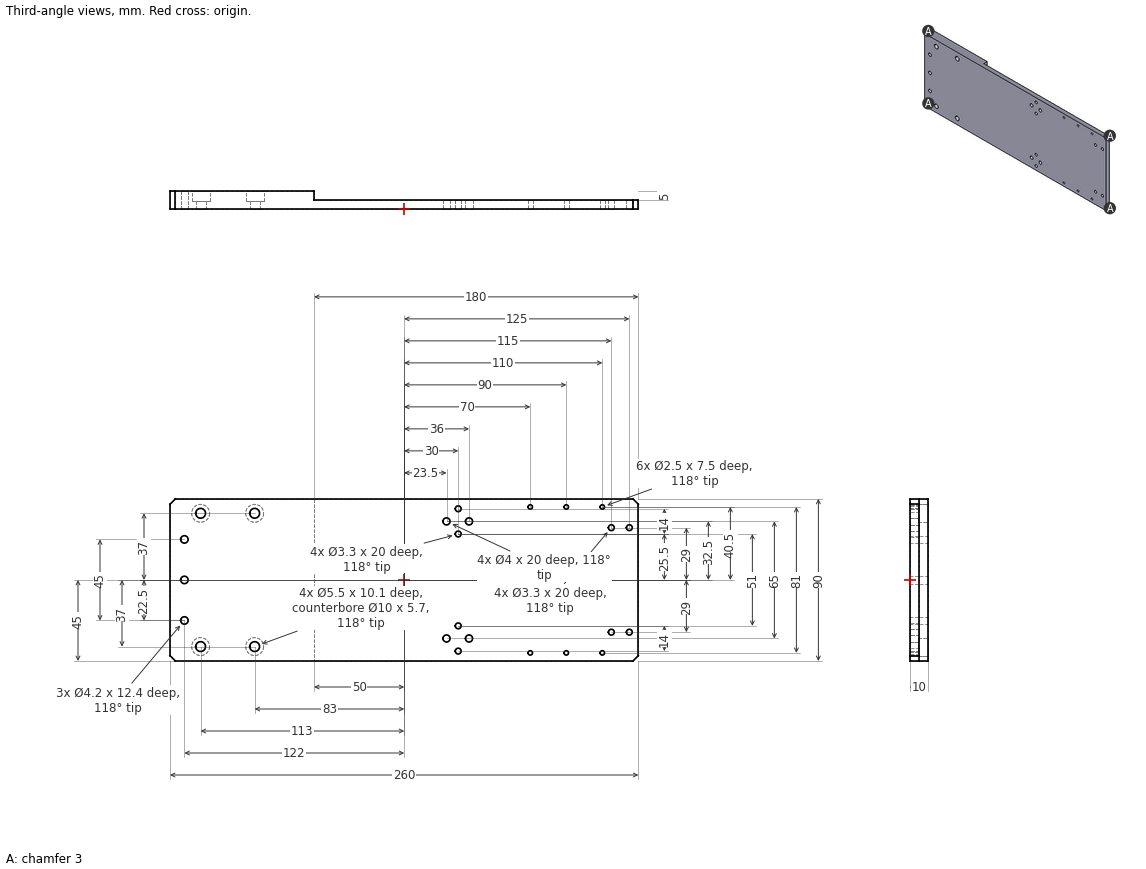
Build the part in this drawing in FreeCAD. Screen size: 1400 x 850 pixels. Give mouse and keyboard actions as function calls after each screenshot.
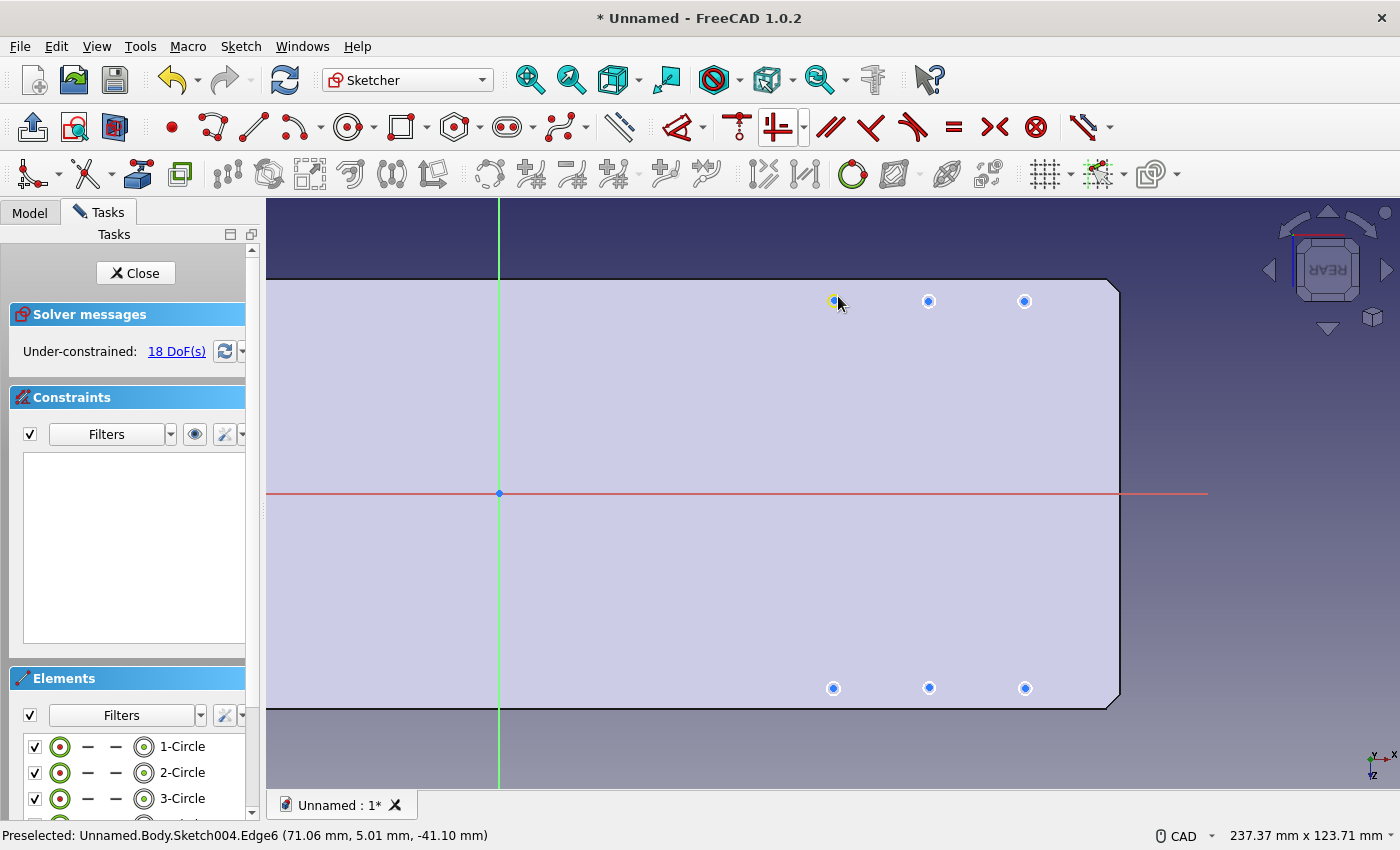
scroll(1030, 684, up, 4)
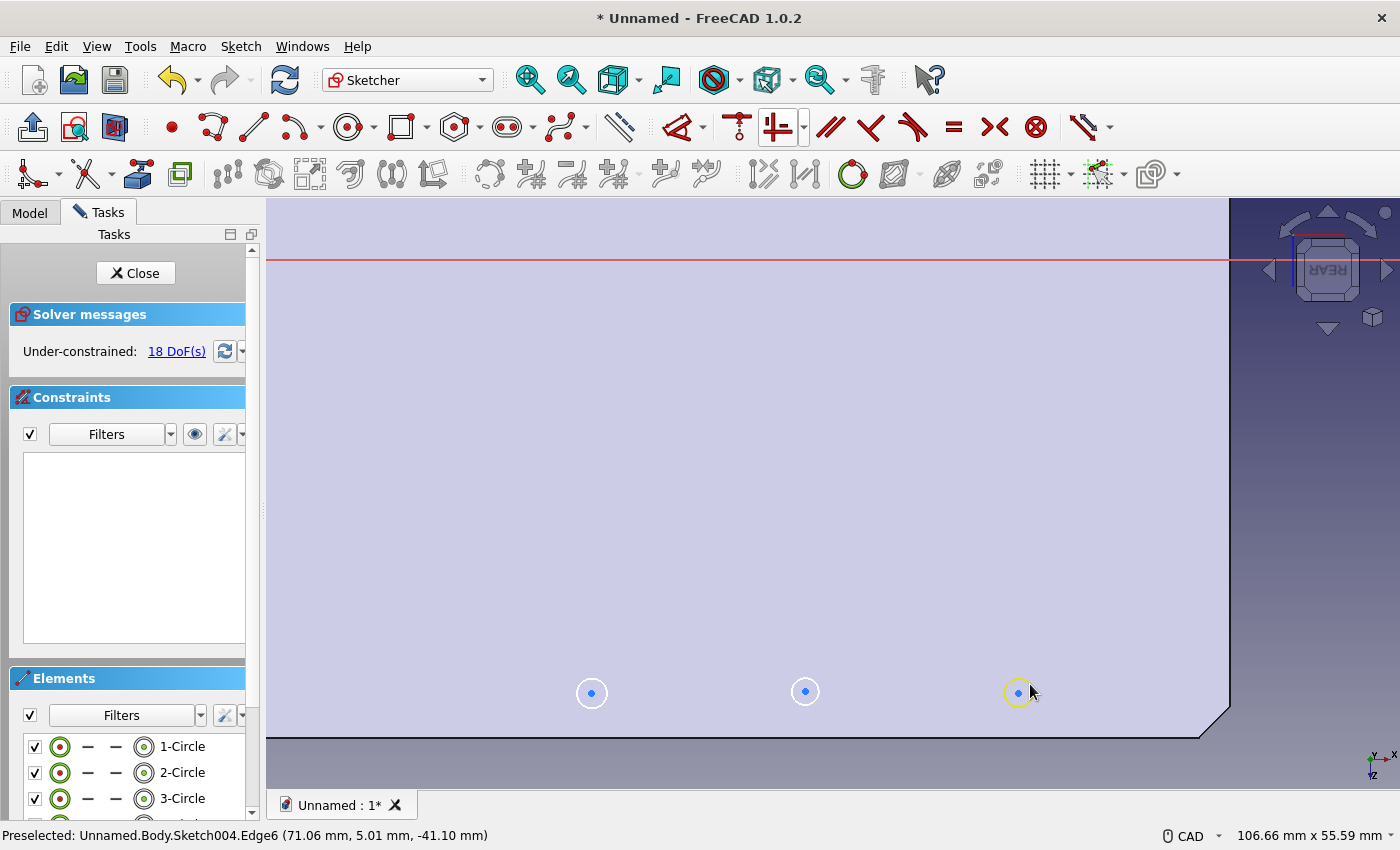
click(1029, 683)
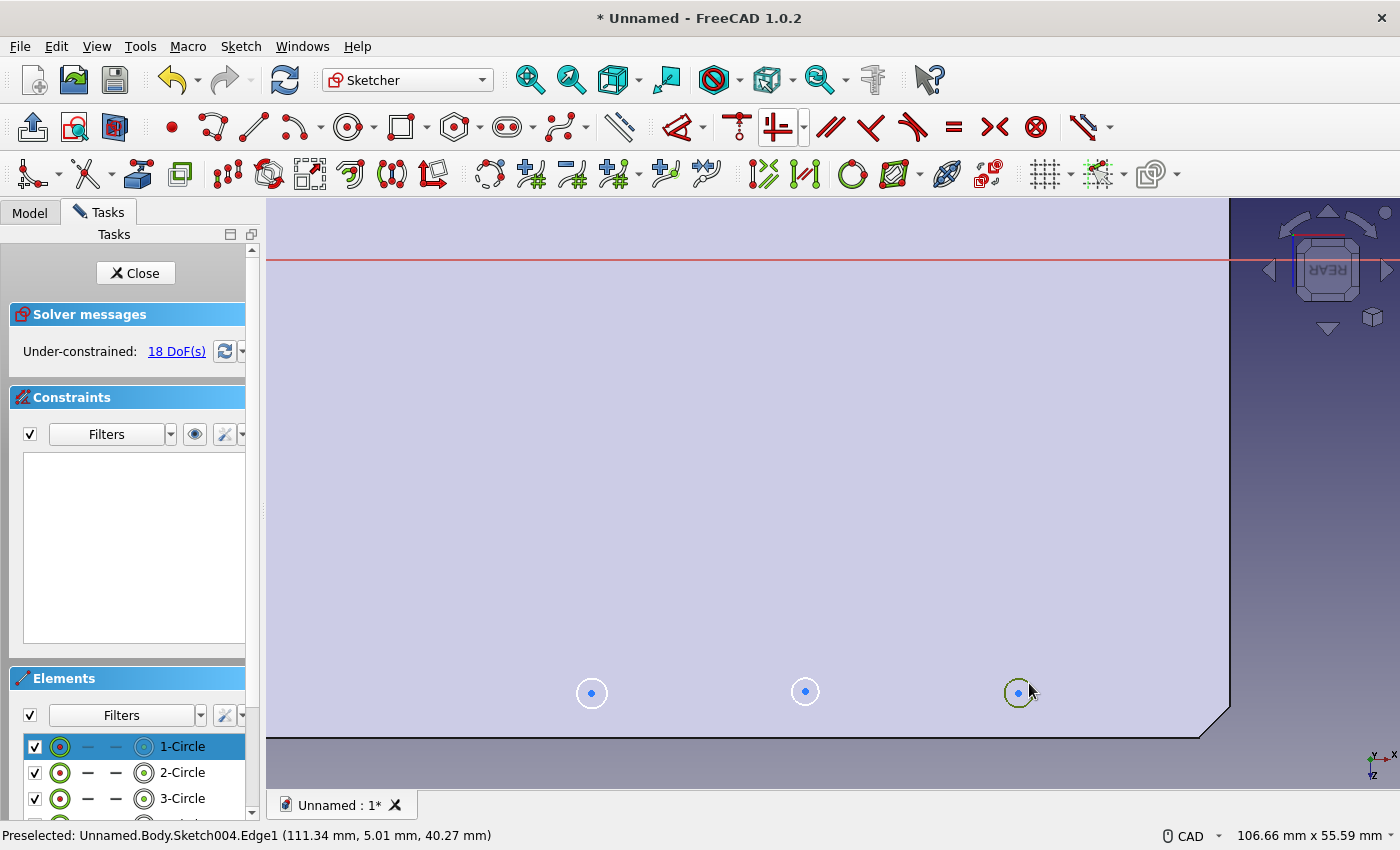
click(815, 682)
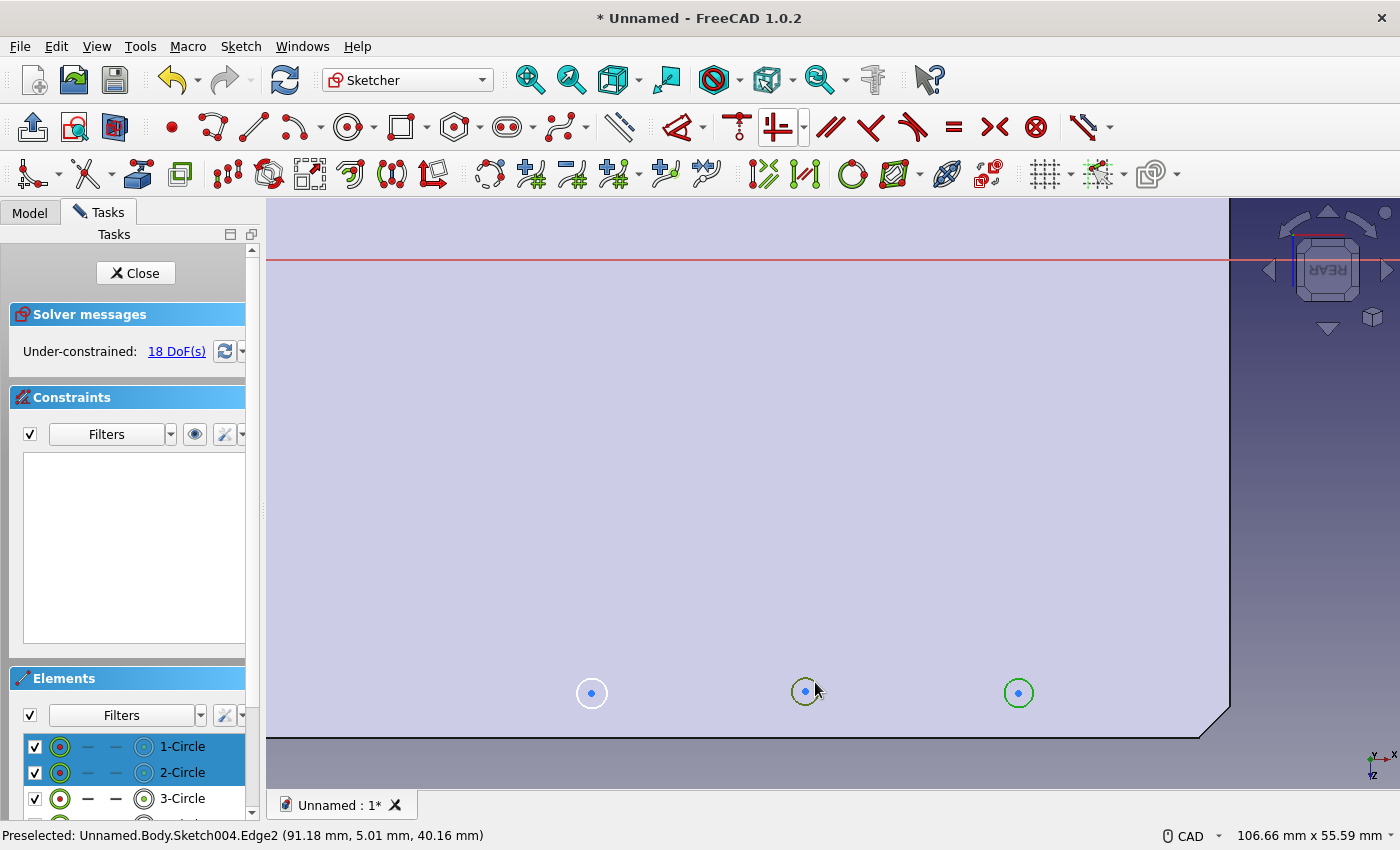
click(602, 683)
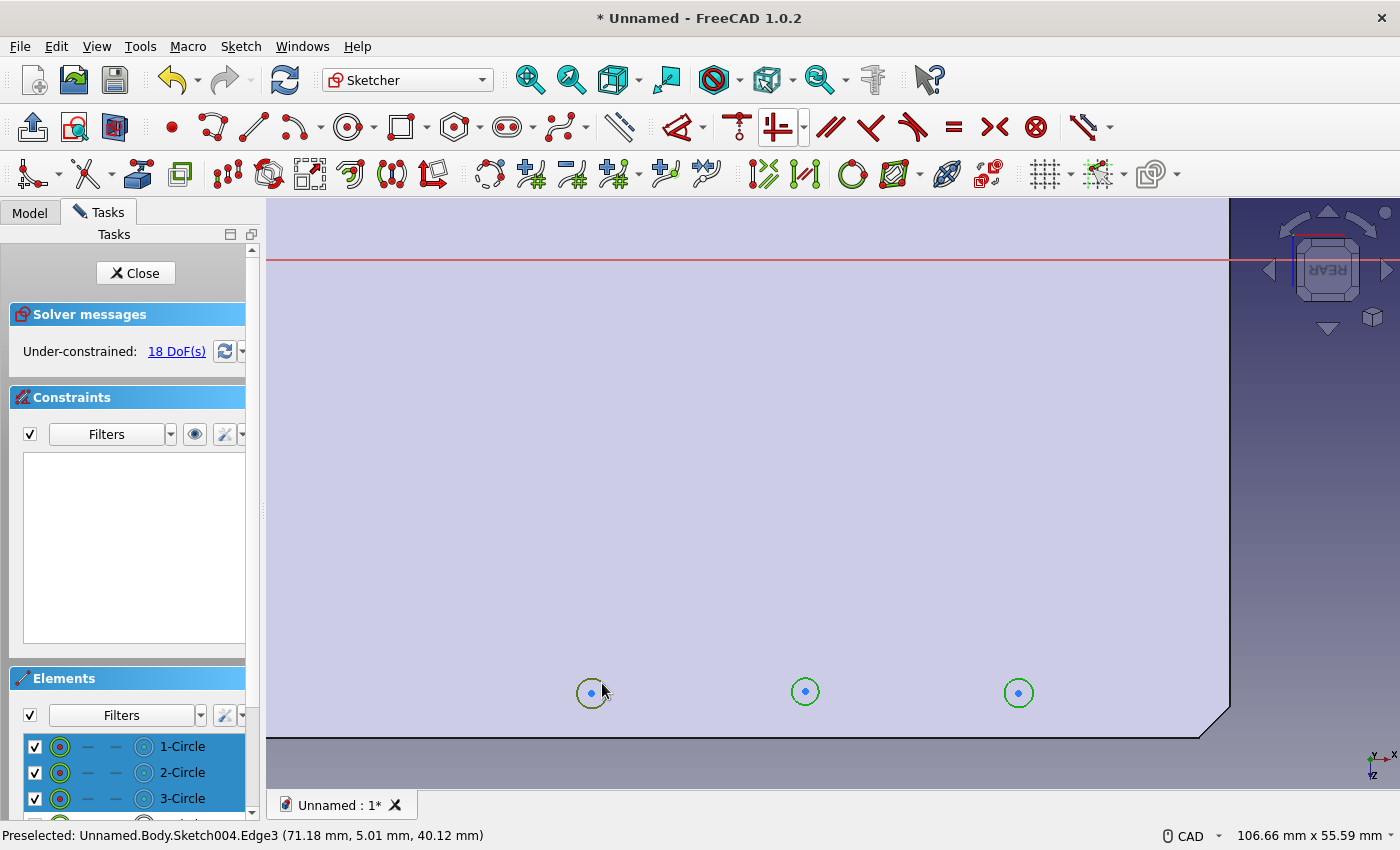
scroll(1030, 684, down, 4)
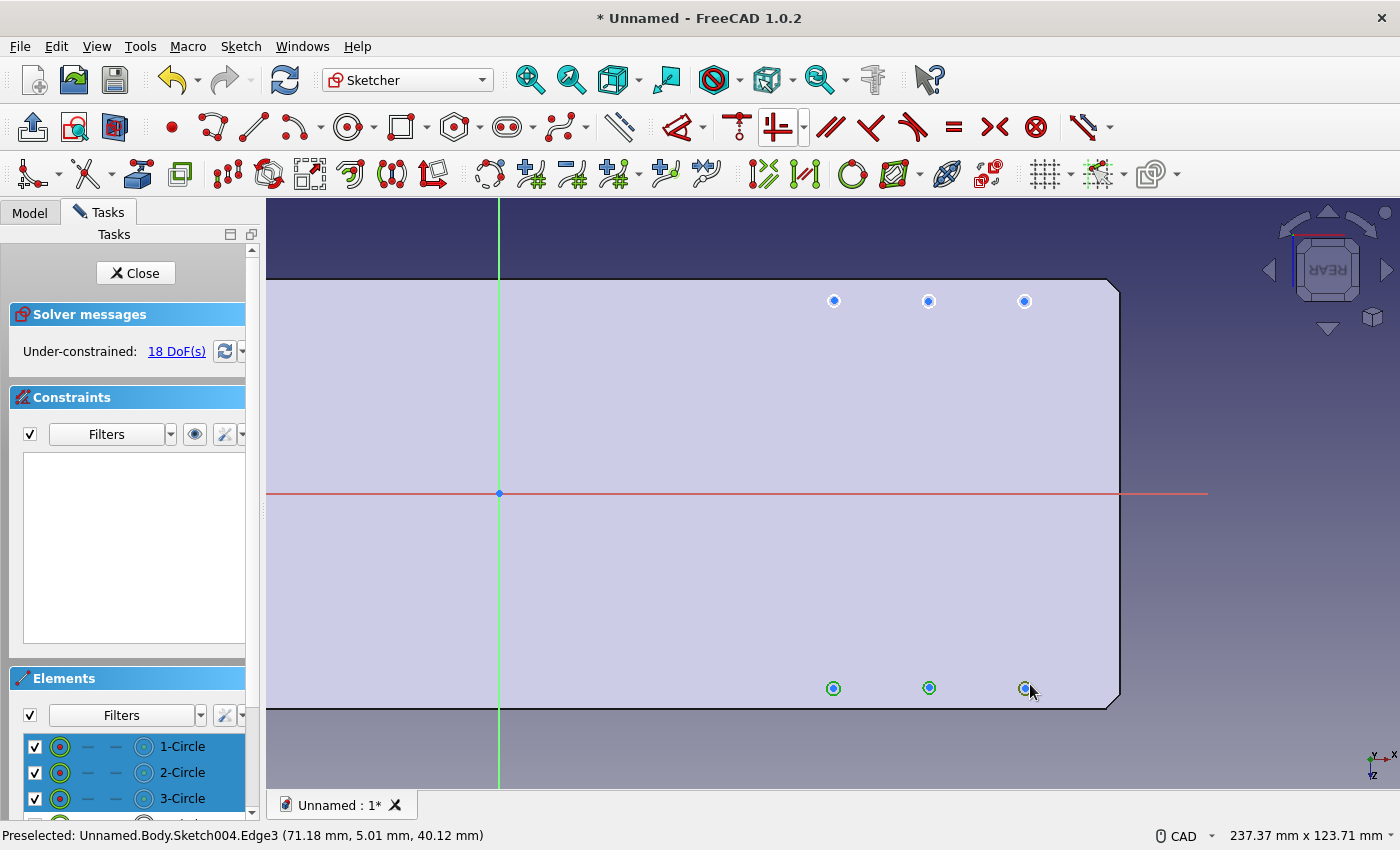
scroll(1029, 297, up, 4)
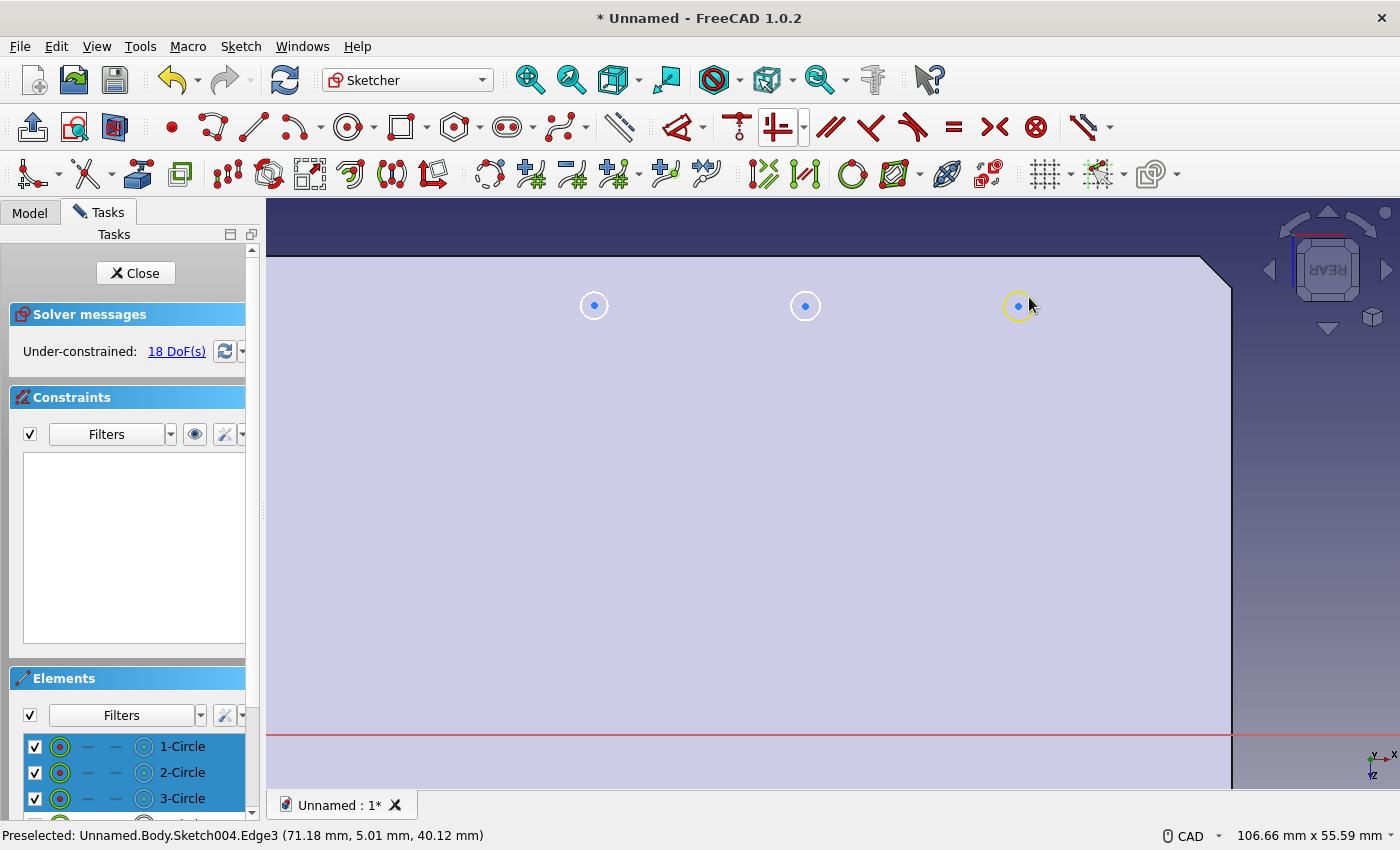
click(1029, 296)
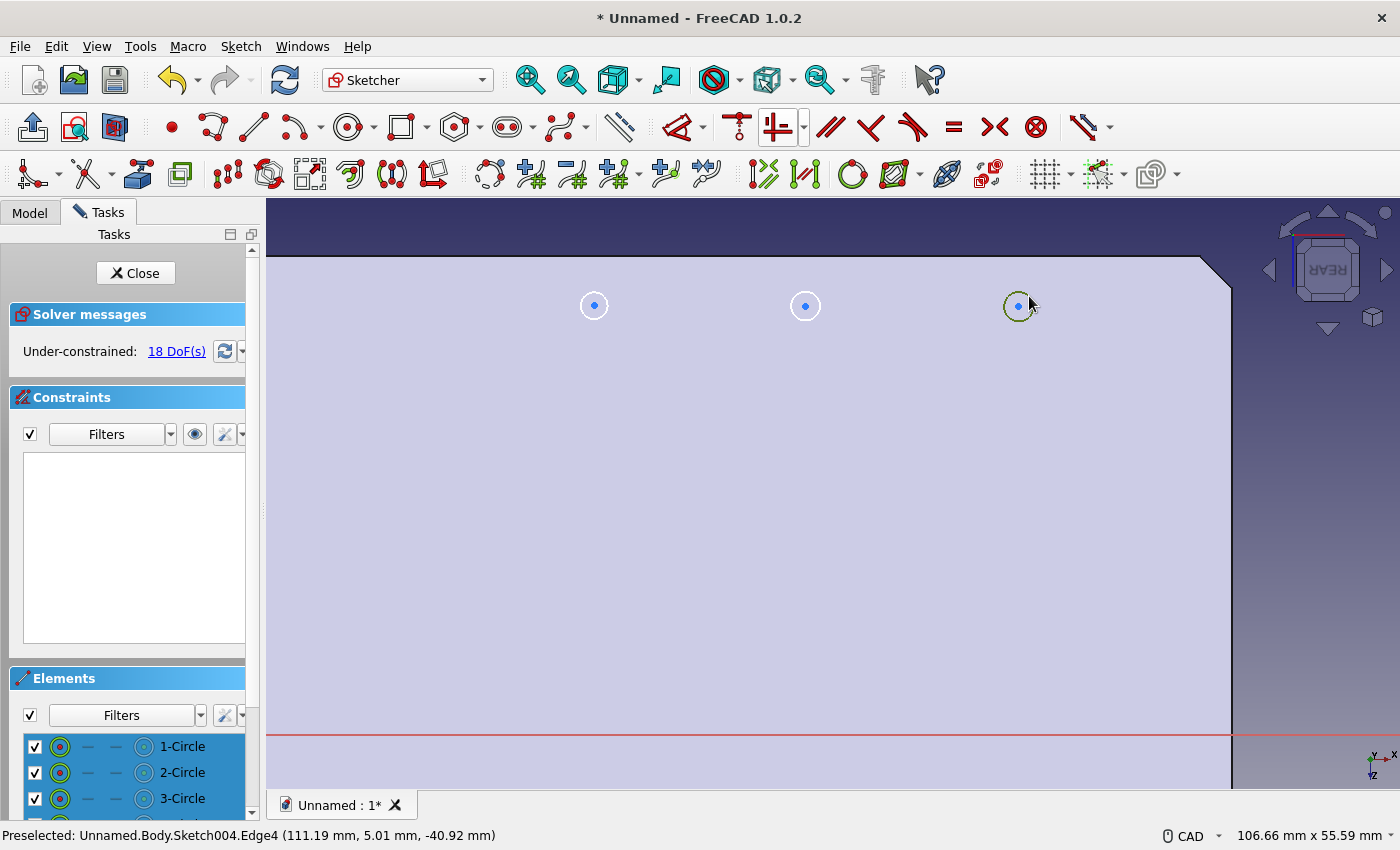
click(816, 296)